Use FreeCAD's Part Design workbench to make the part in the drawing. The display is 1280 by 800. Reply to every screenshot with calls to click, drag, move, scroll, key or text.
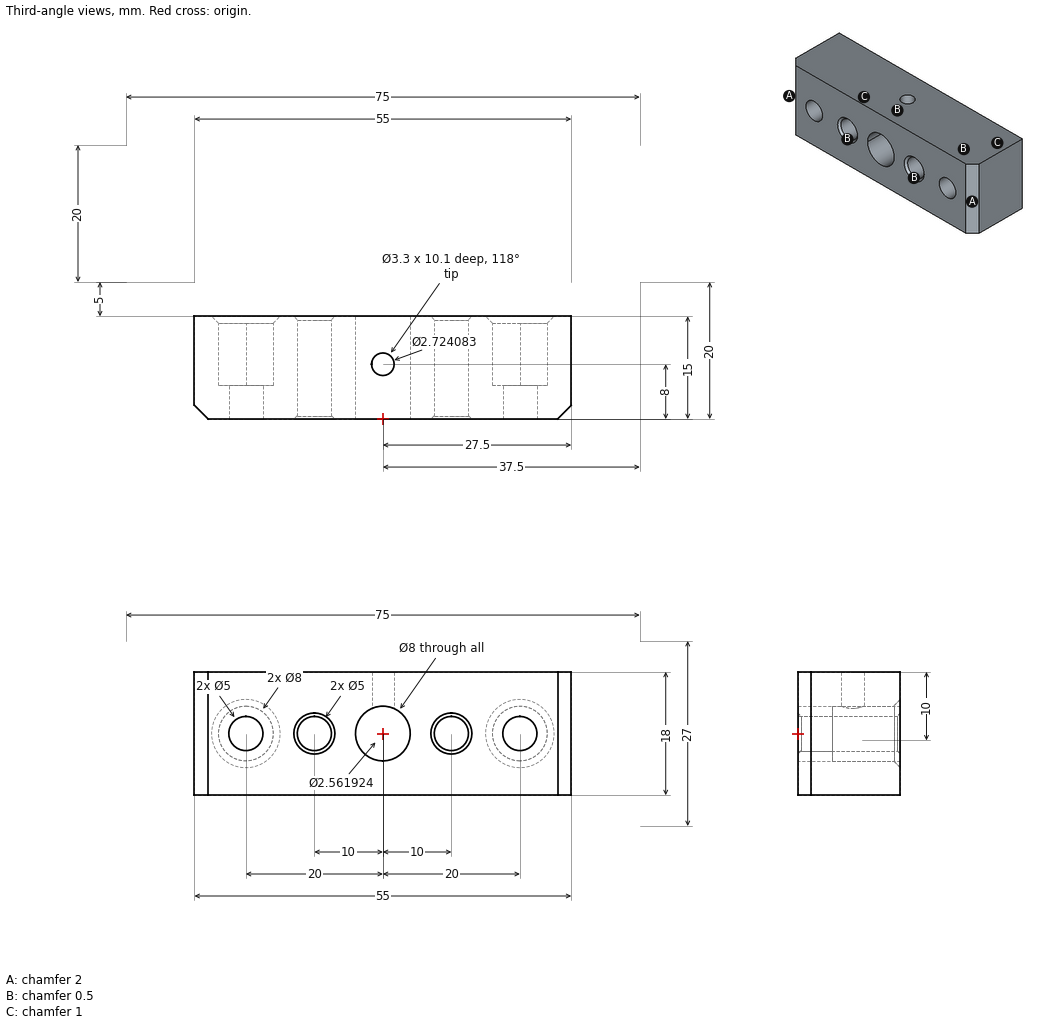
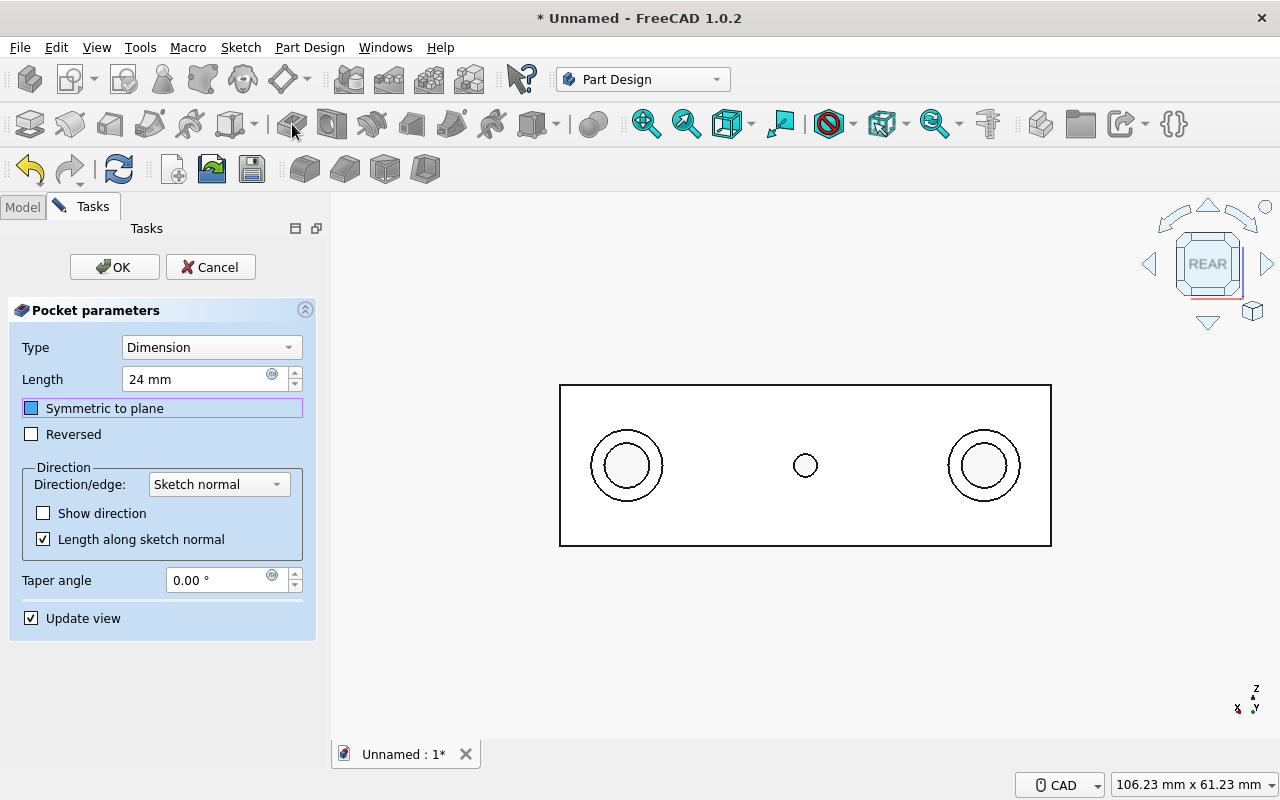
click(115, 267)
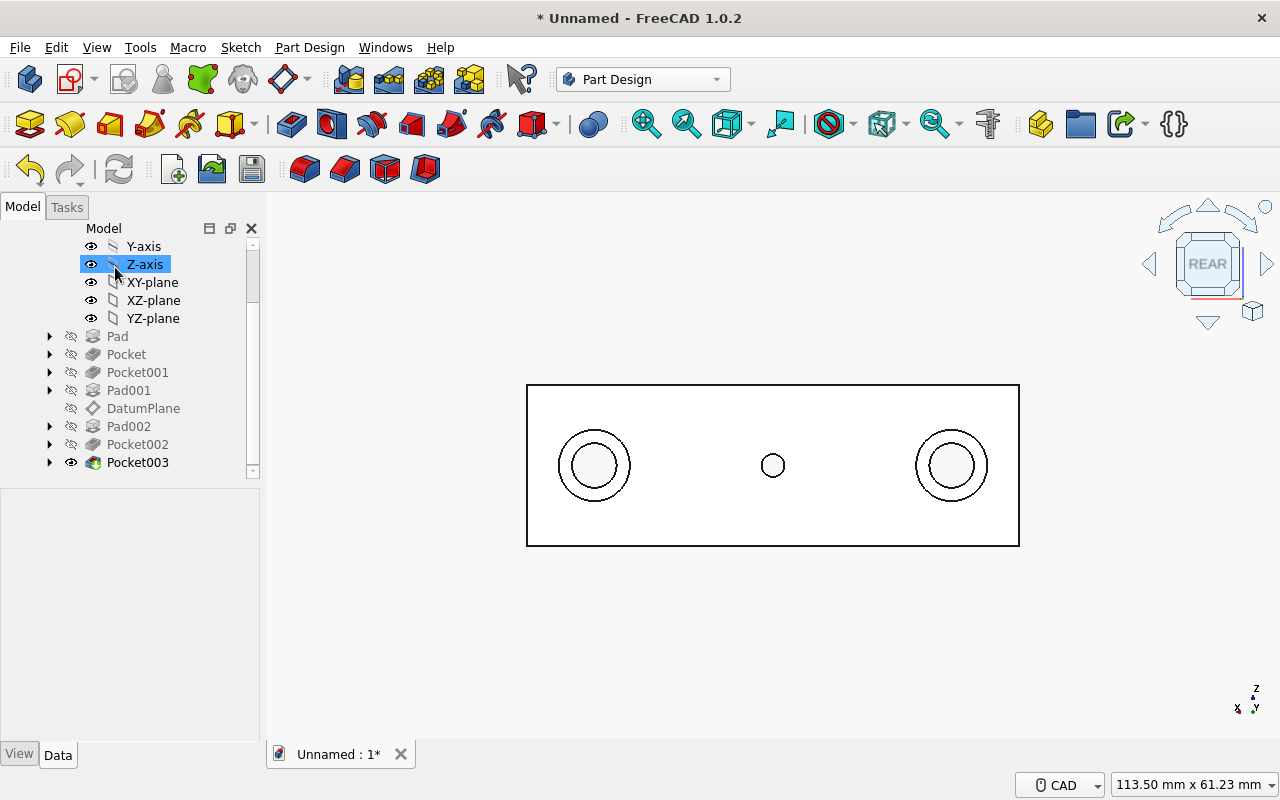
click(703, 465)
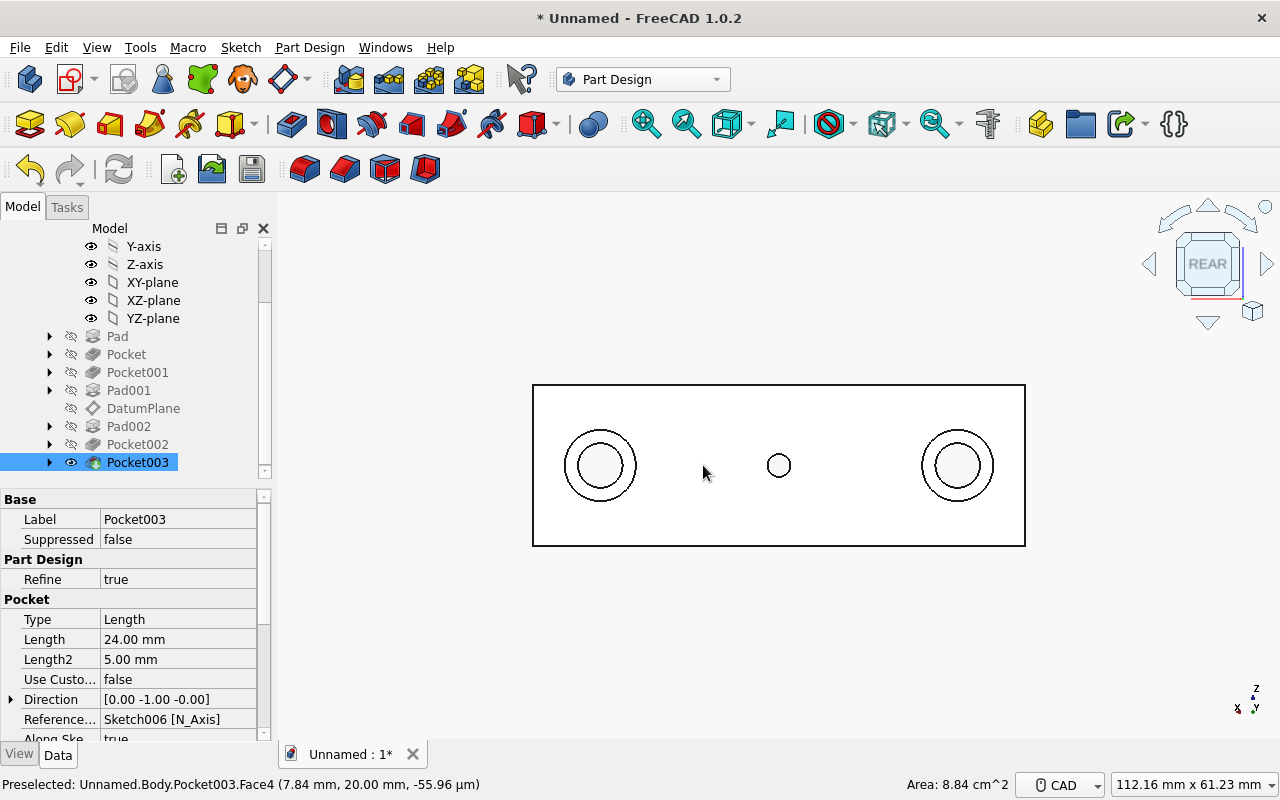
click(70, 80)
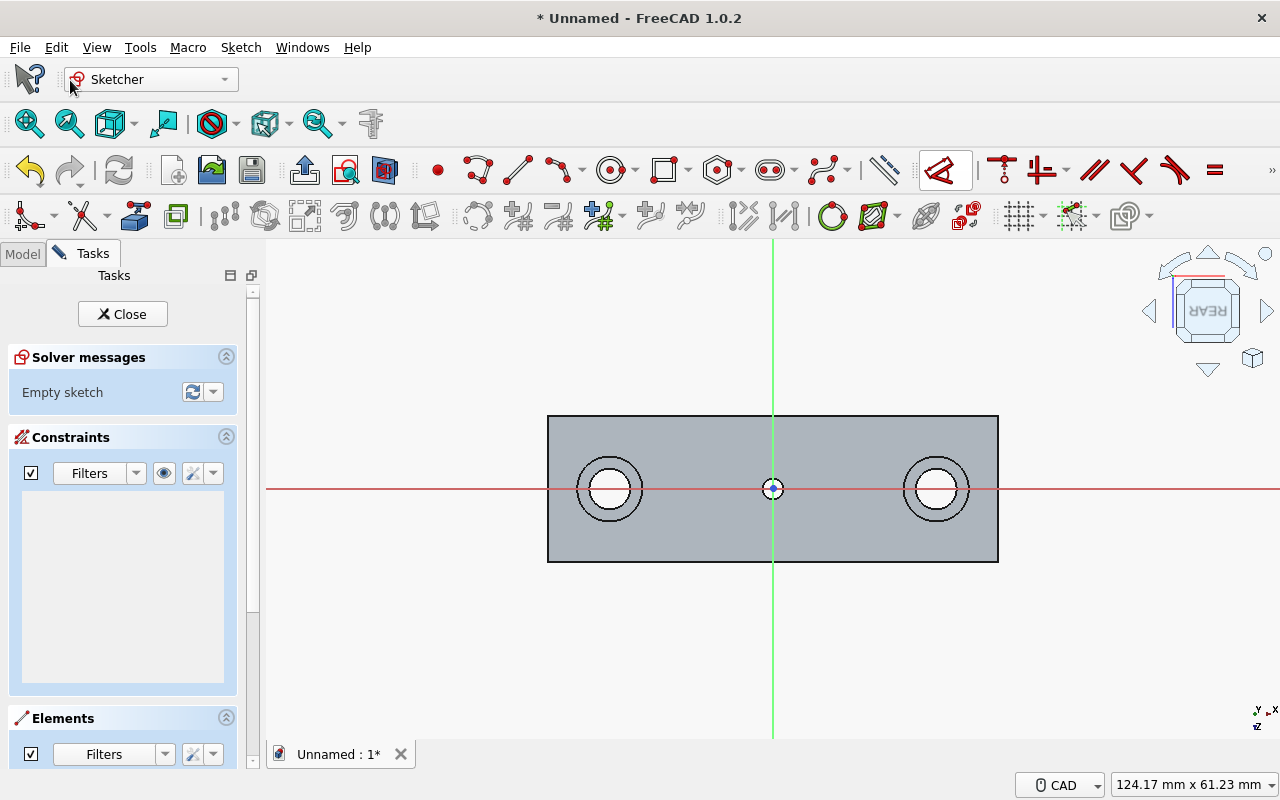
scroll(790, 489, up, 8)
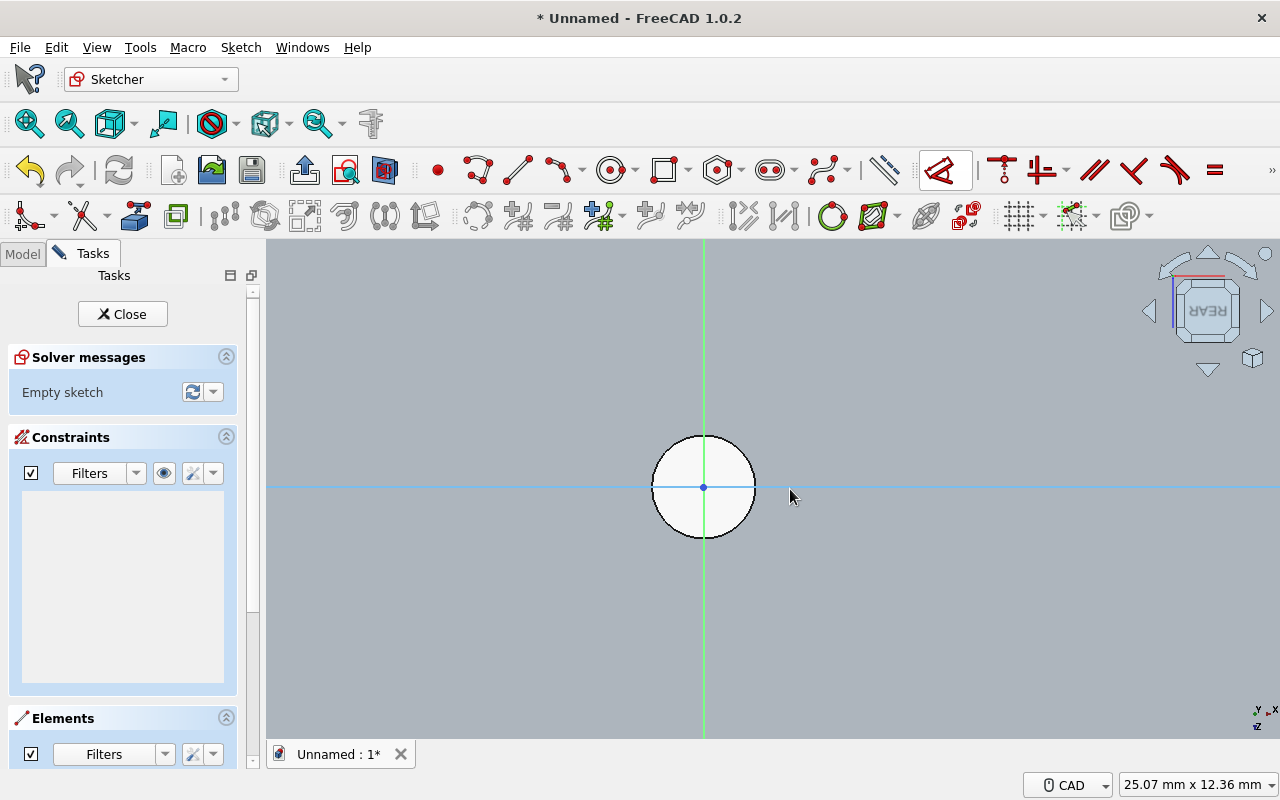
click(612, 170)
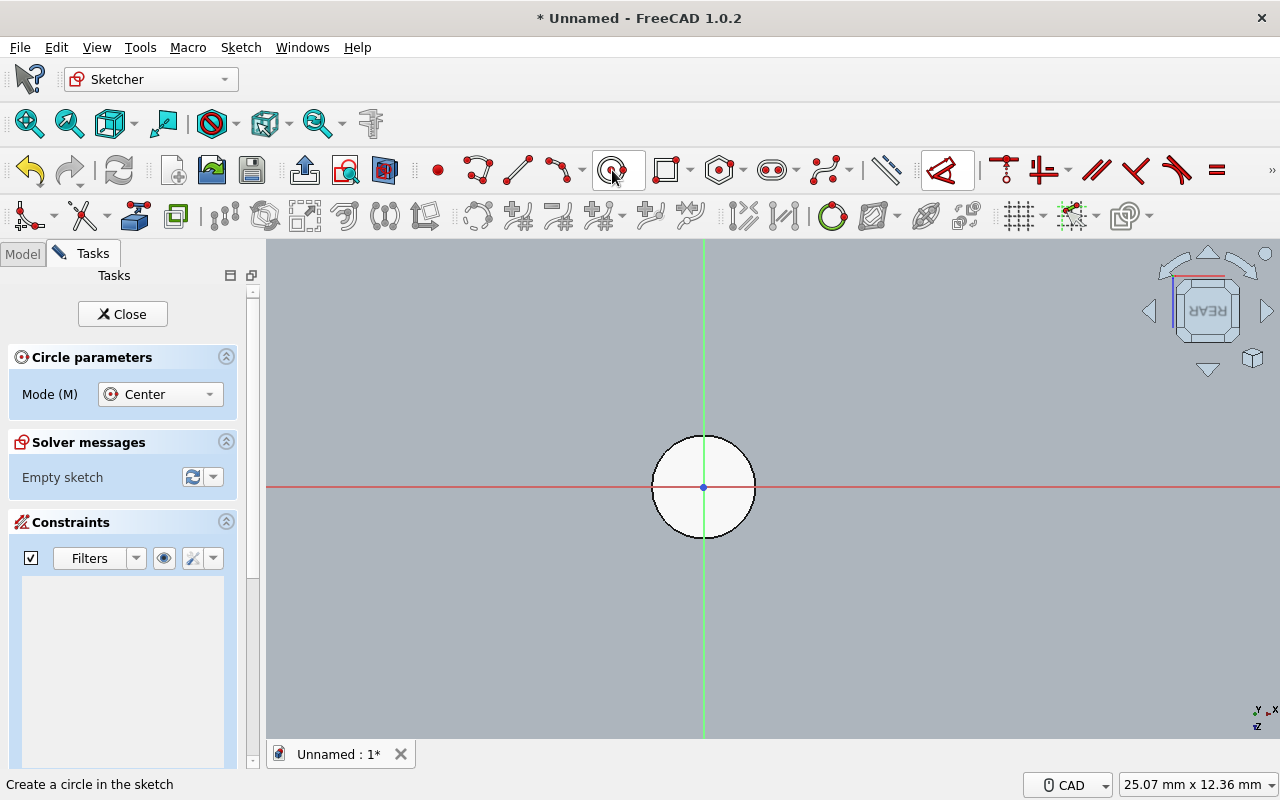
click(704, 487)
move(818, 373)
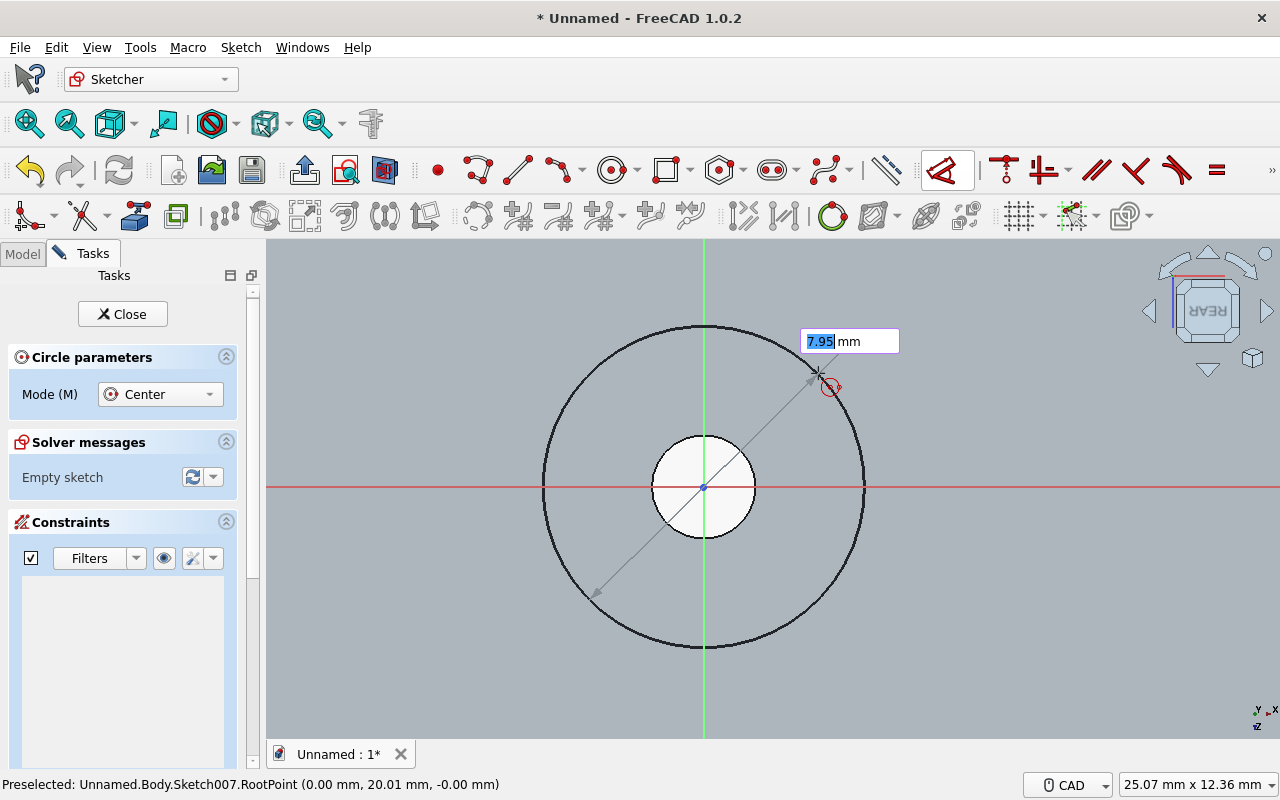
text(8)
key(Return)
key(Escape)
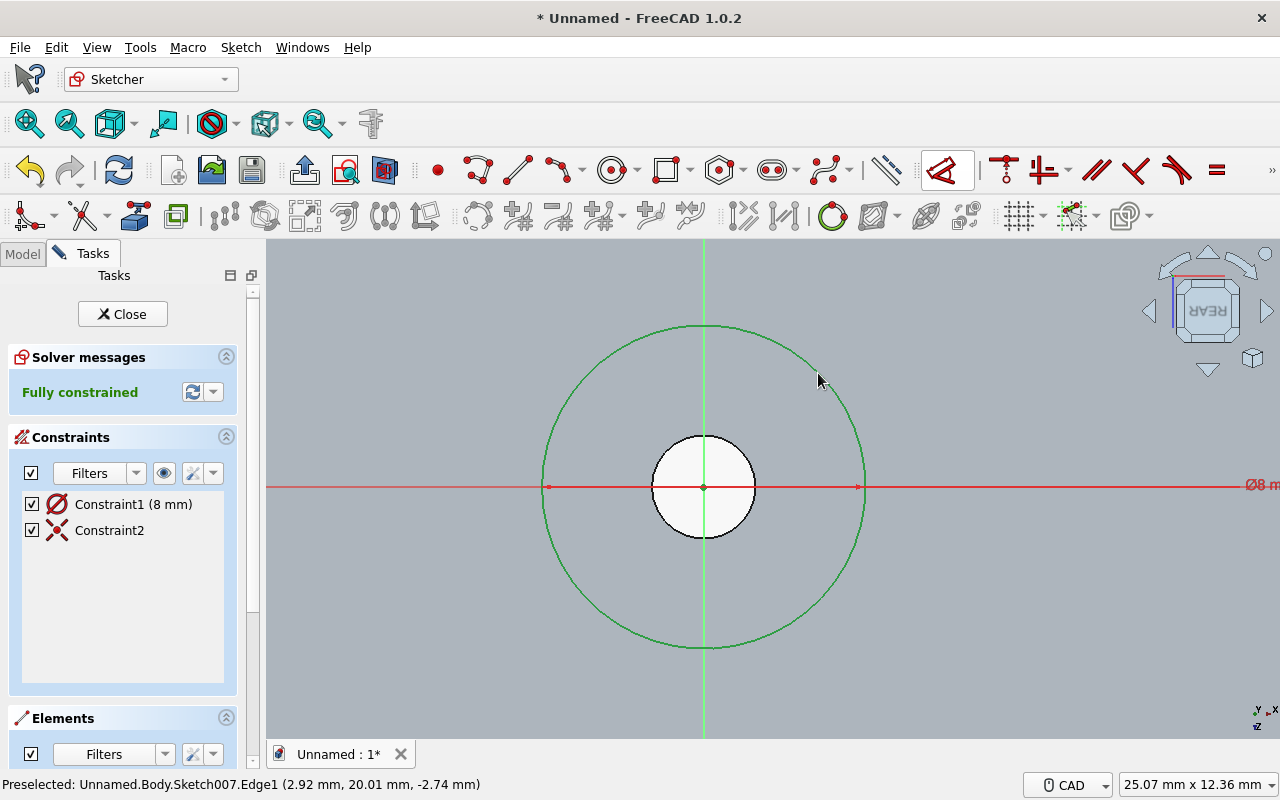
click(123, 314)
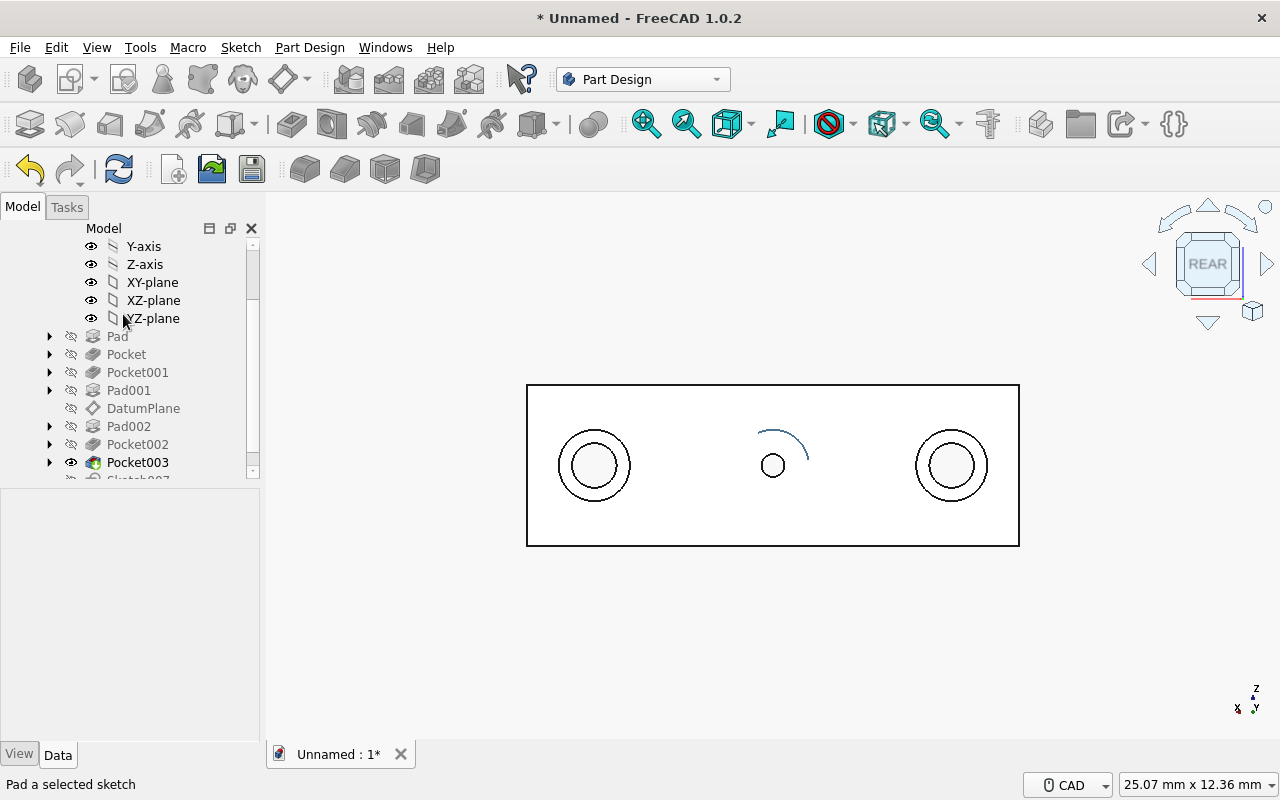
click(332, 124)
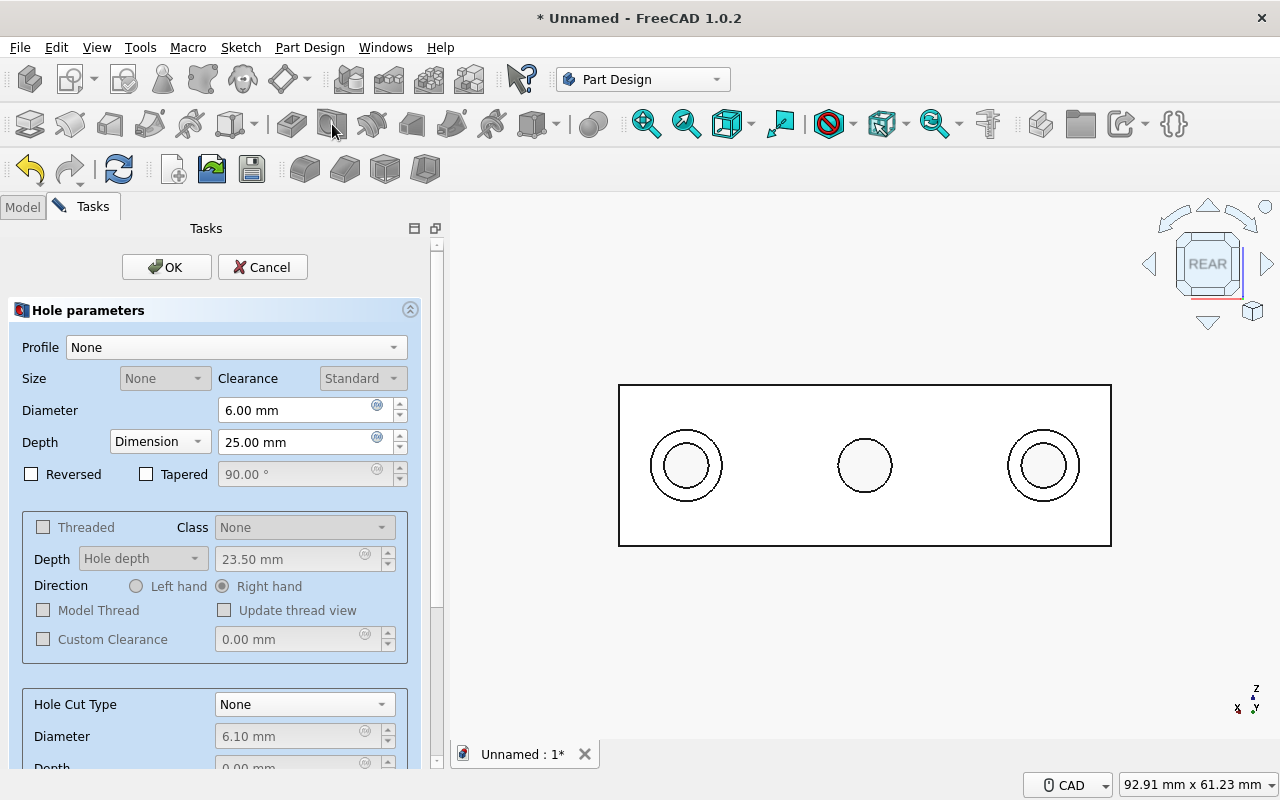
triple_click(305, 410)